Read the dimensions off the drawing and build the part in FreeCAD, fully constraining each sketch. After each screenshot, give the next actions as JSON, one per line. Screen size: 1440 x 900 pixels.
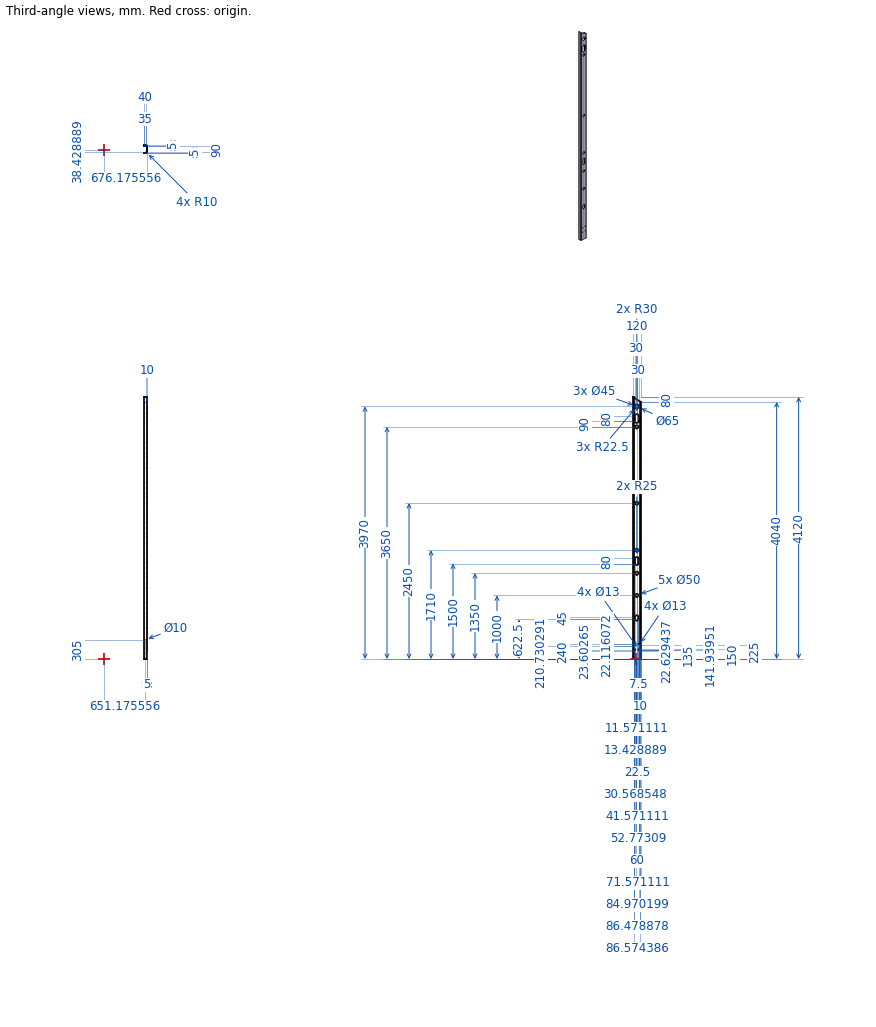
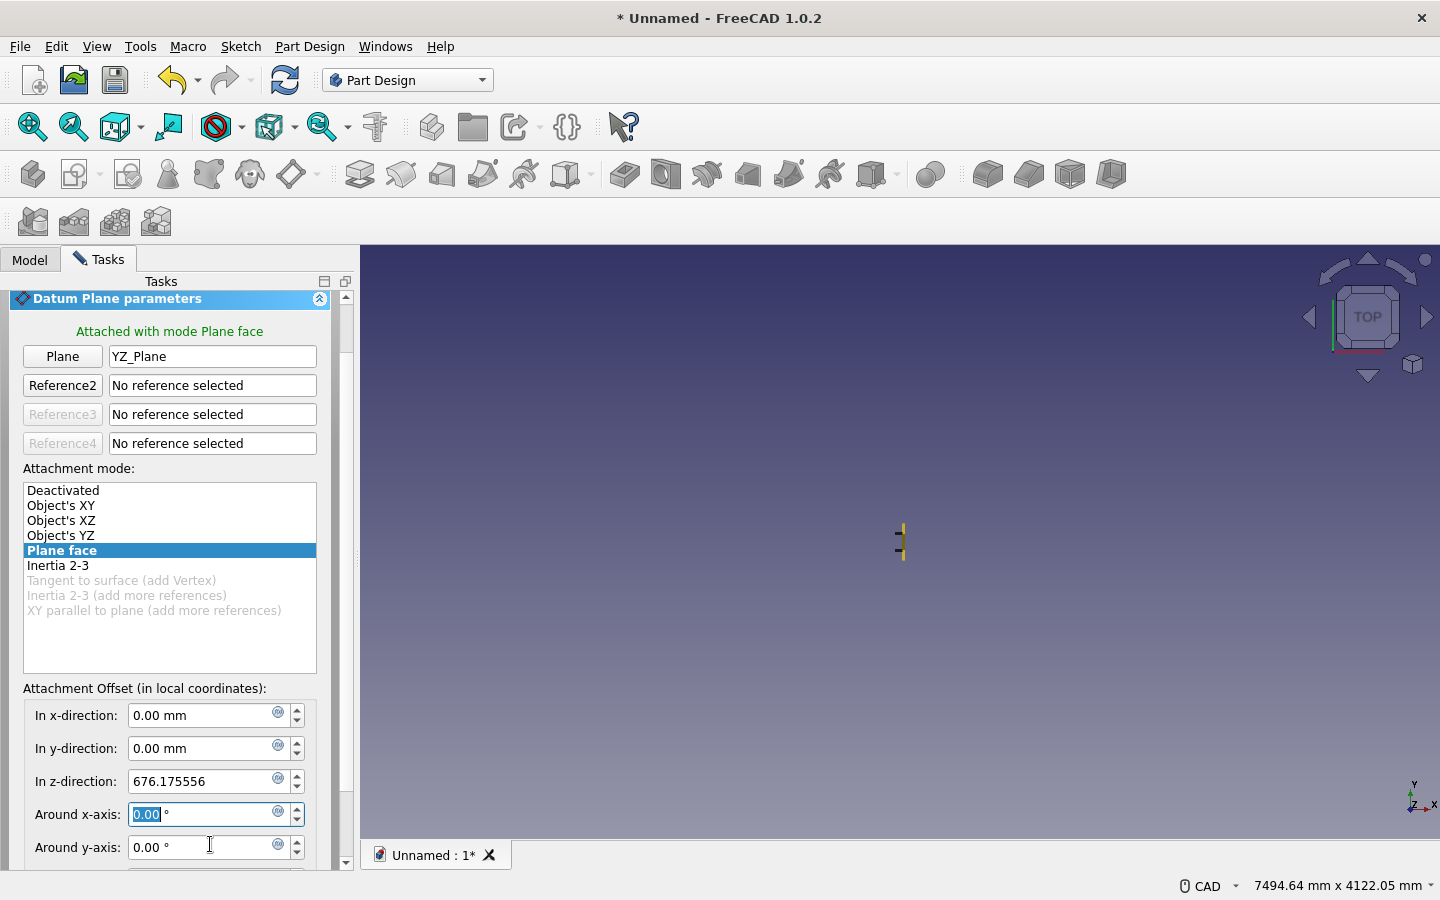
{"action": "scroll", "coordinate": [346, 580], "scroll_direction": "up", "scroll_amount": 2}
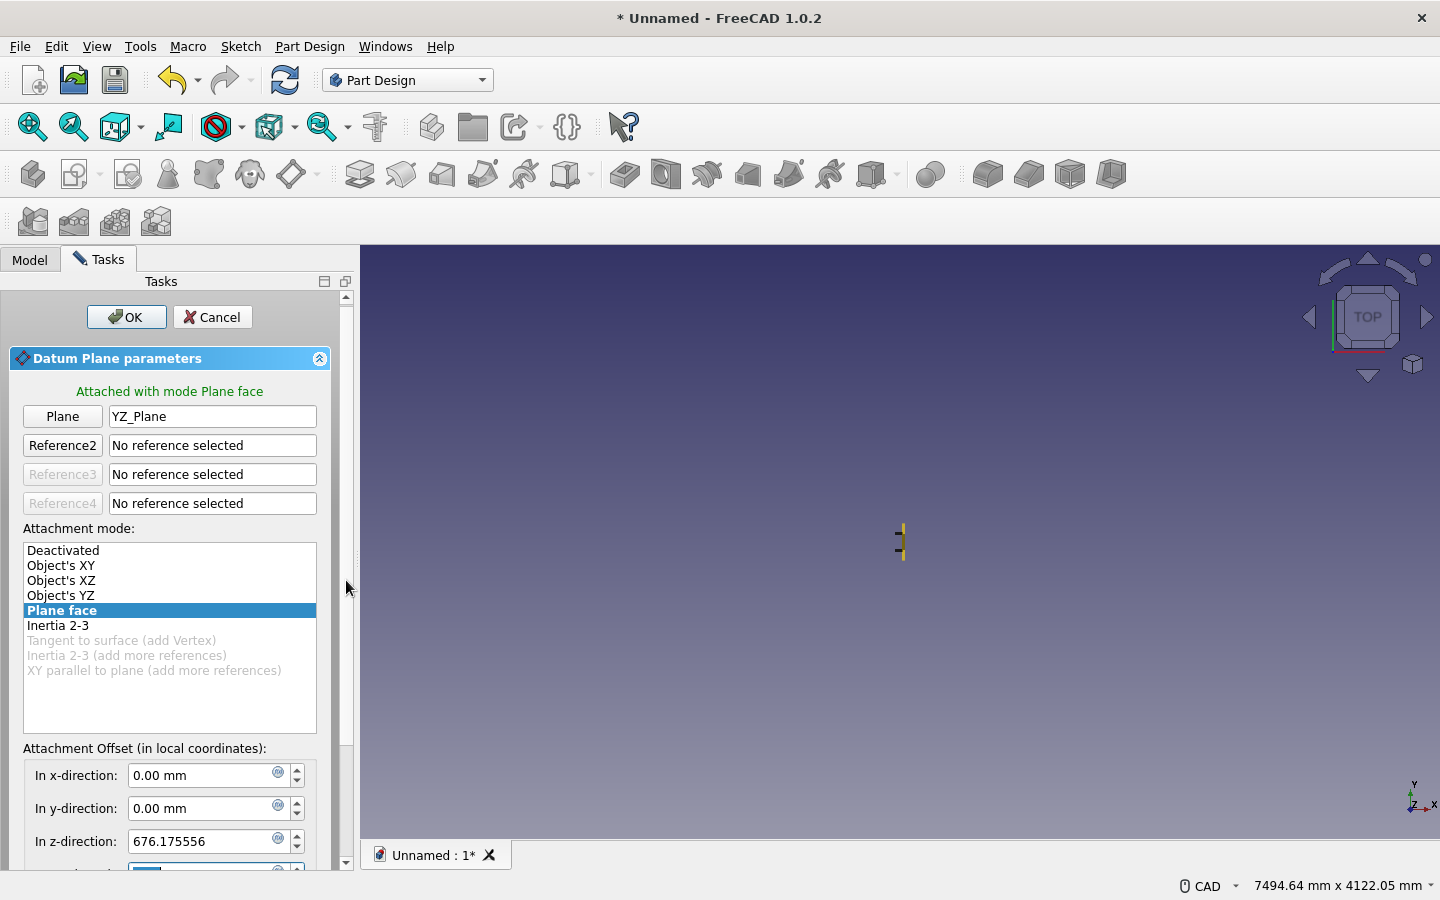
{"action": "left_click", "coordinate": [127, 320]}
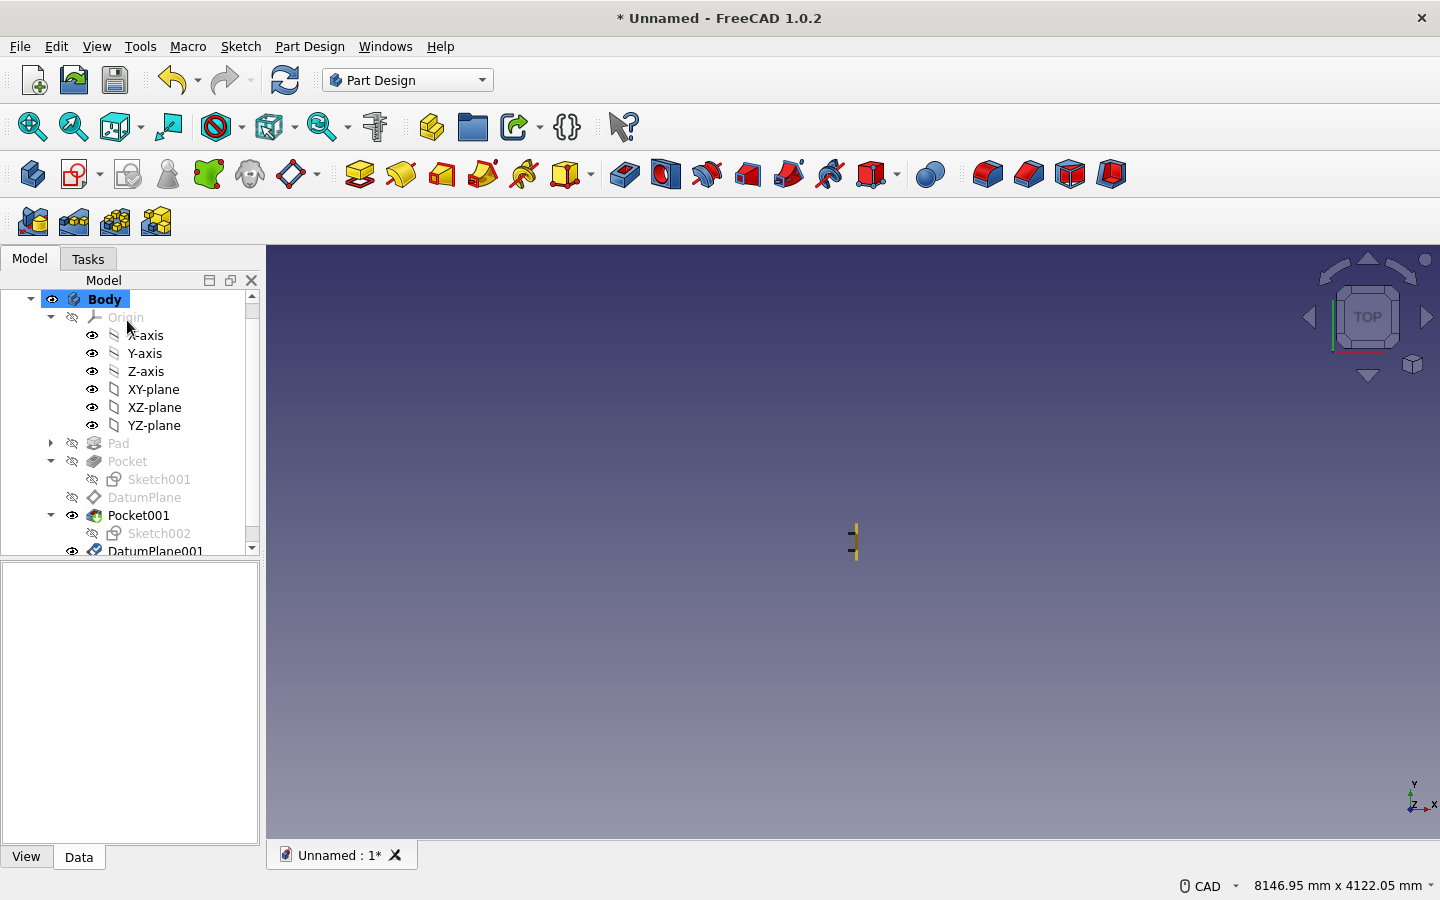
{"action": "left_click", "coordinate": [117, 551]}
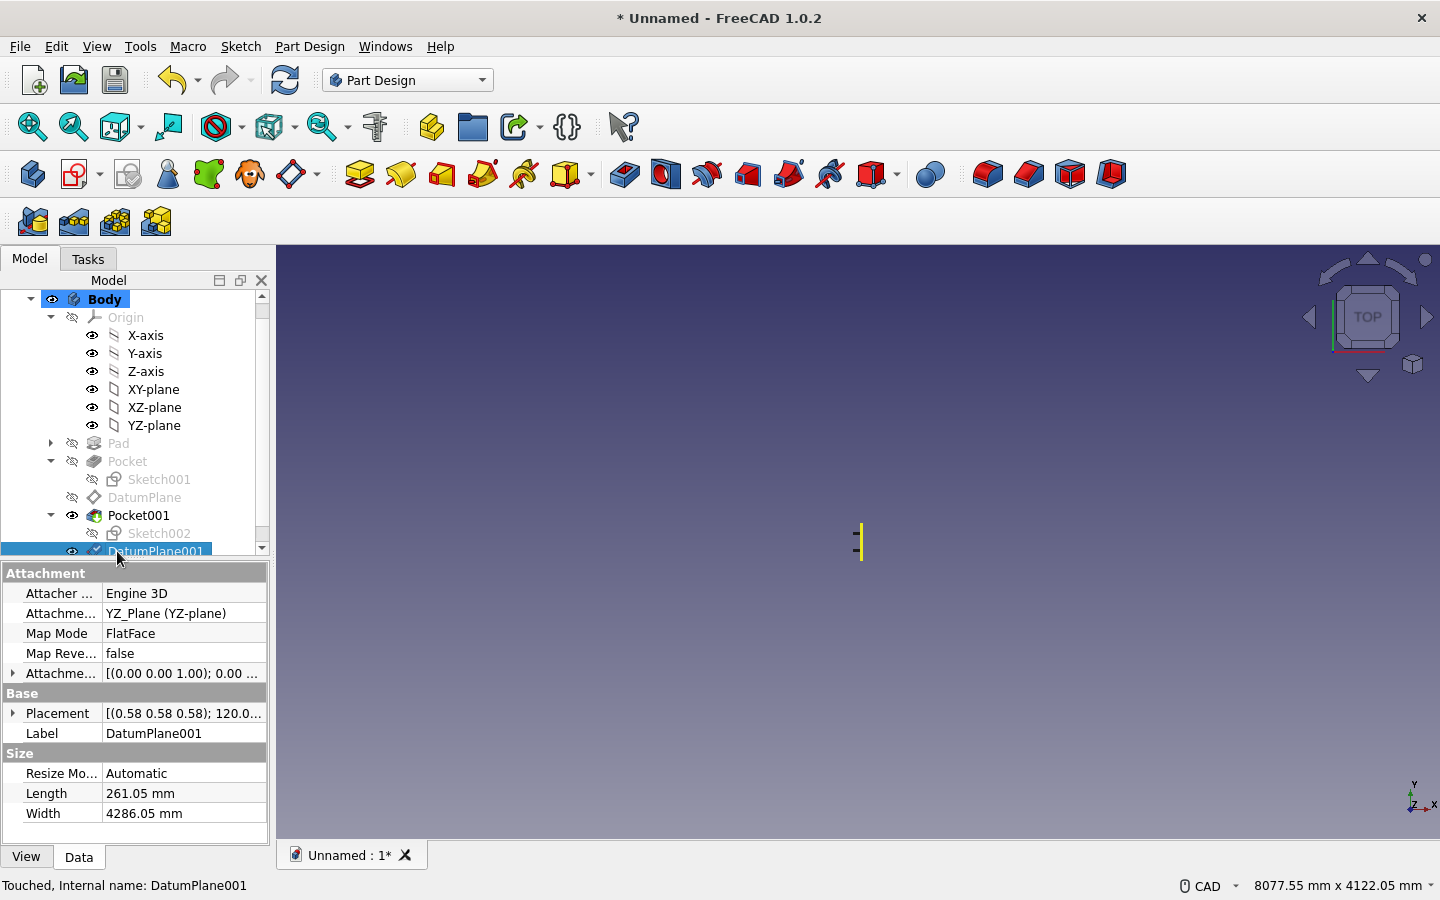
{"action": "left_click", "coordinate": [74, 174]}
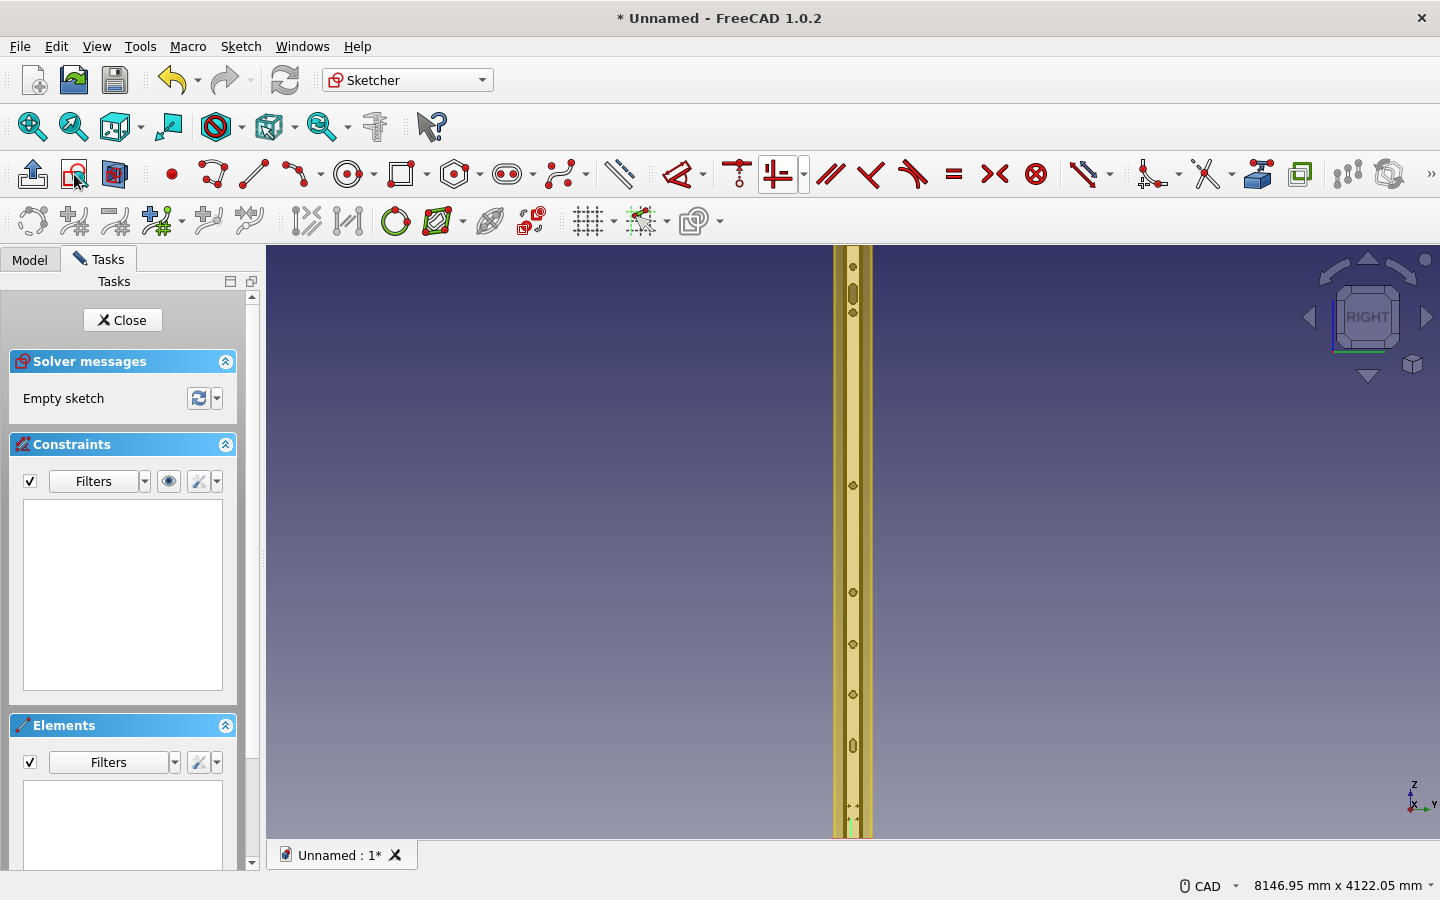
{"action": "scroll", "coordinate": [857, 621], "scroll_direction": "up", "scroll_amount": 15}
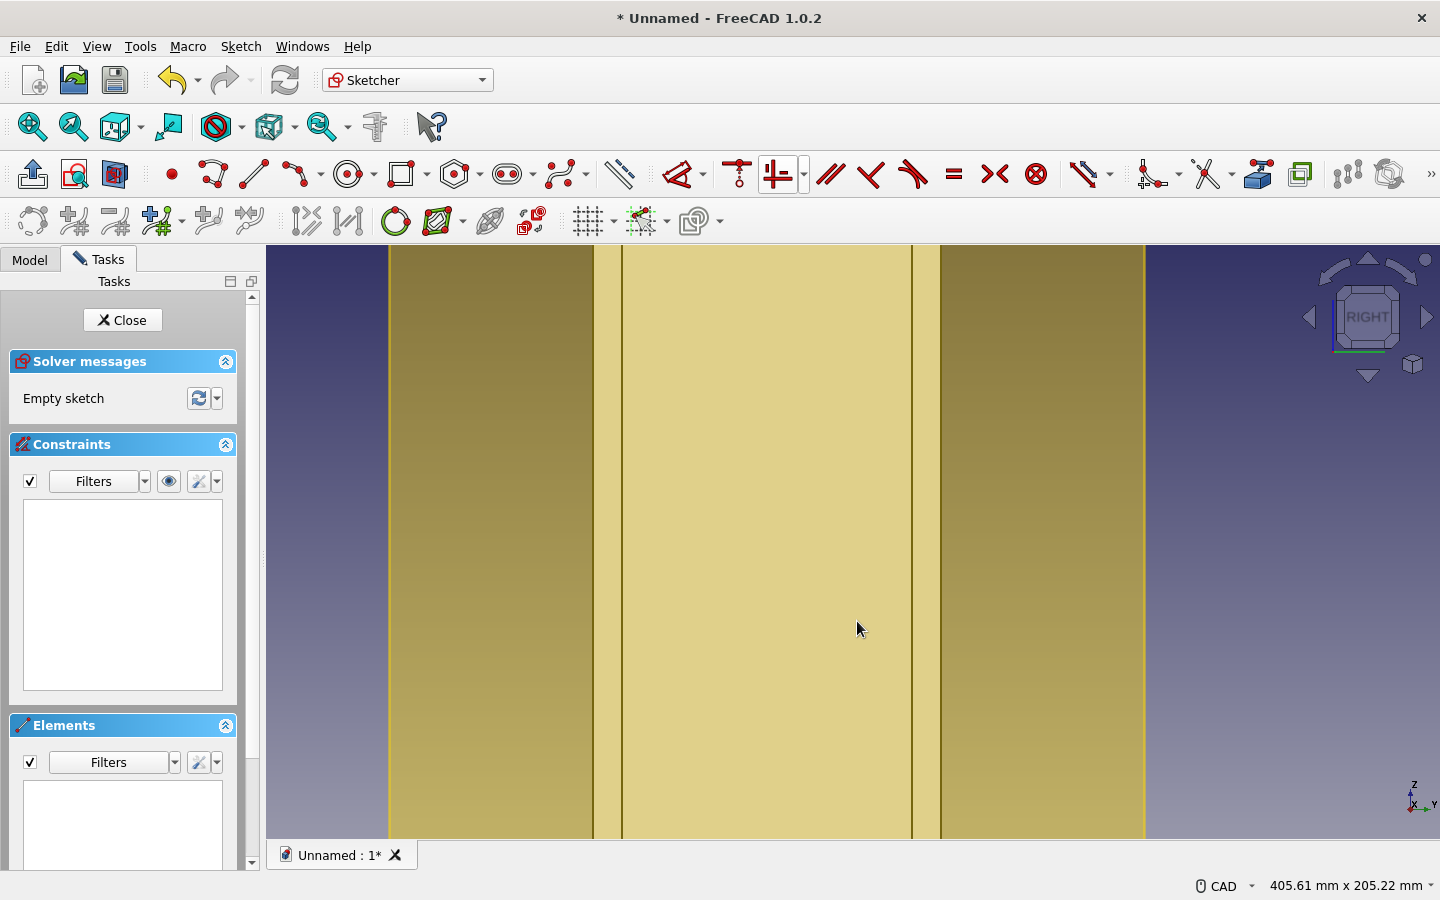
{"action": "key", "text": "g s"}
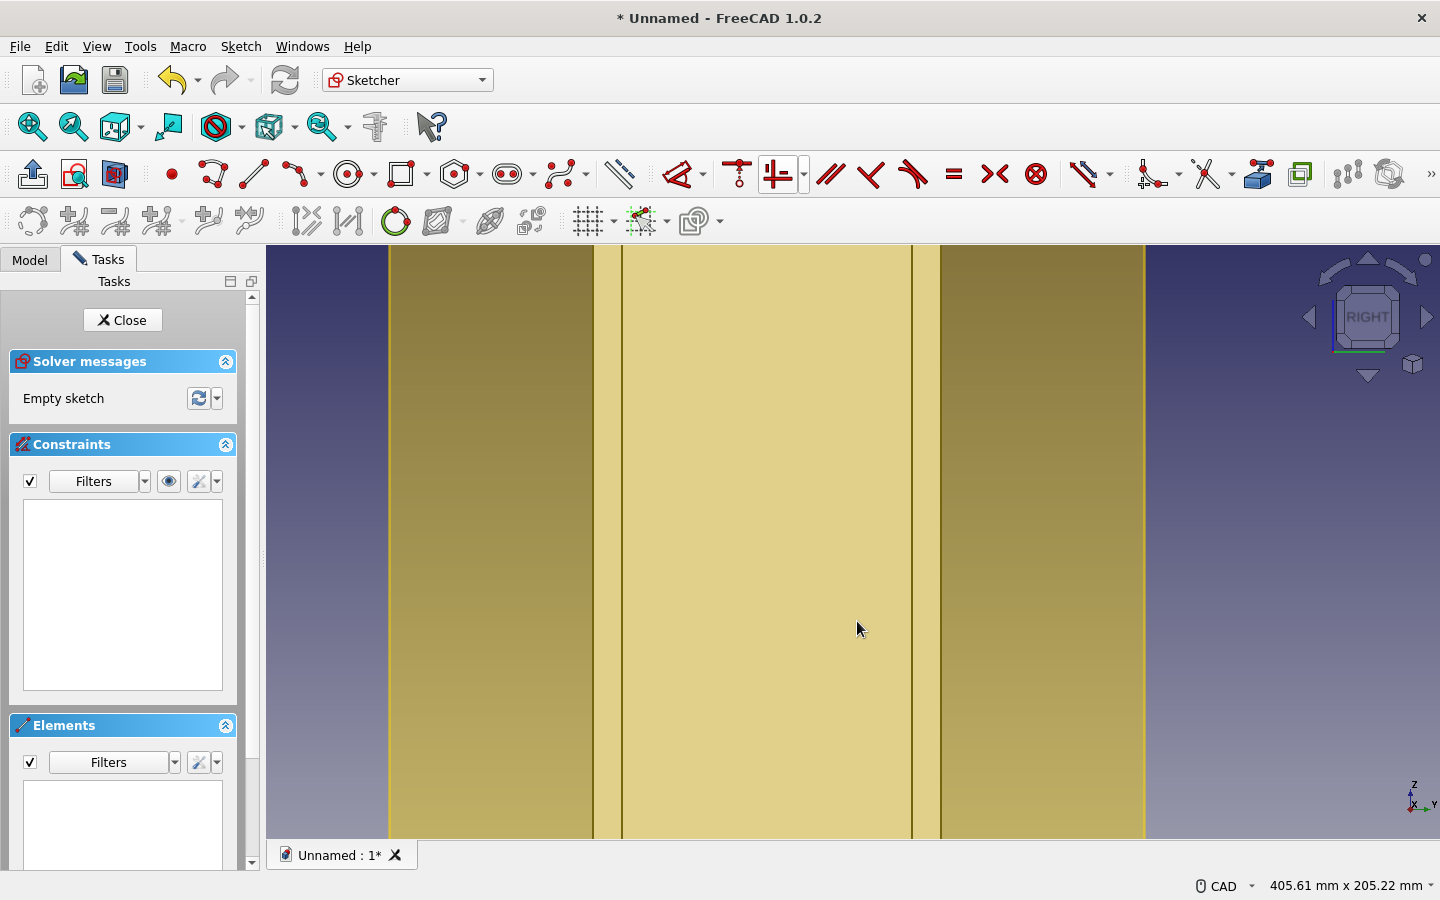
{"action": "left_click", "coordinate": [767, 643]}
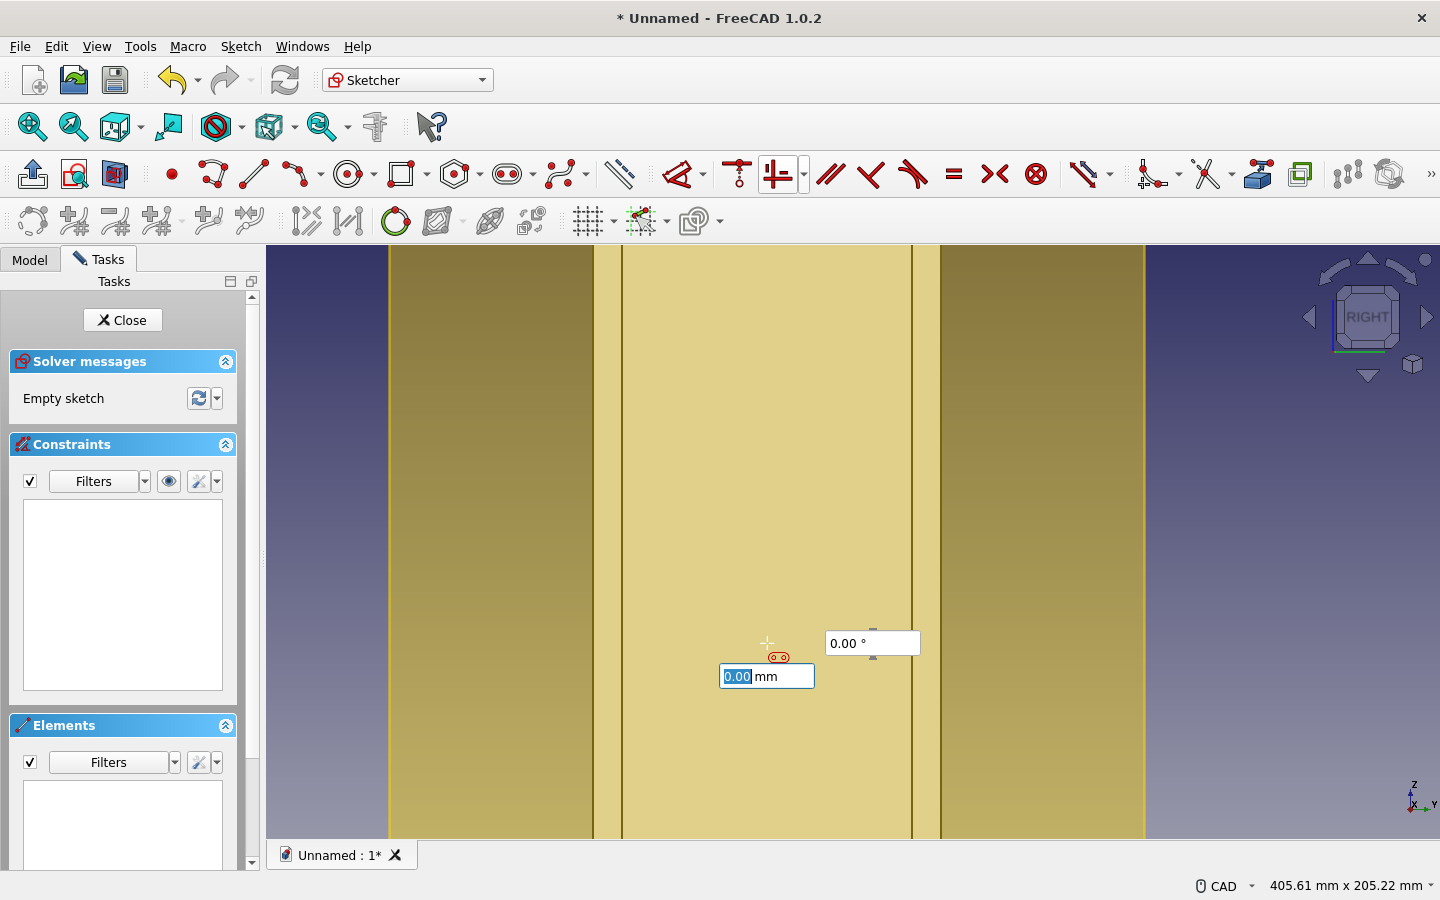
{"action": "left_click", "coordinate": [767, 411]}